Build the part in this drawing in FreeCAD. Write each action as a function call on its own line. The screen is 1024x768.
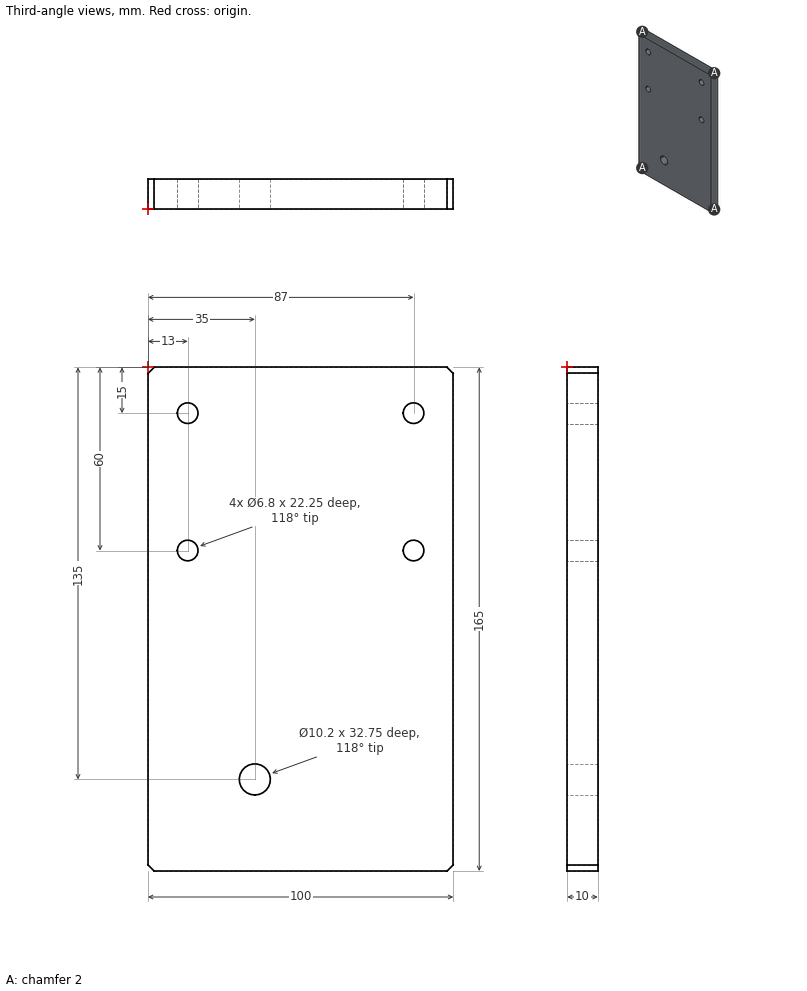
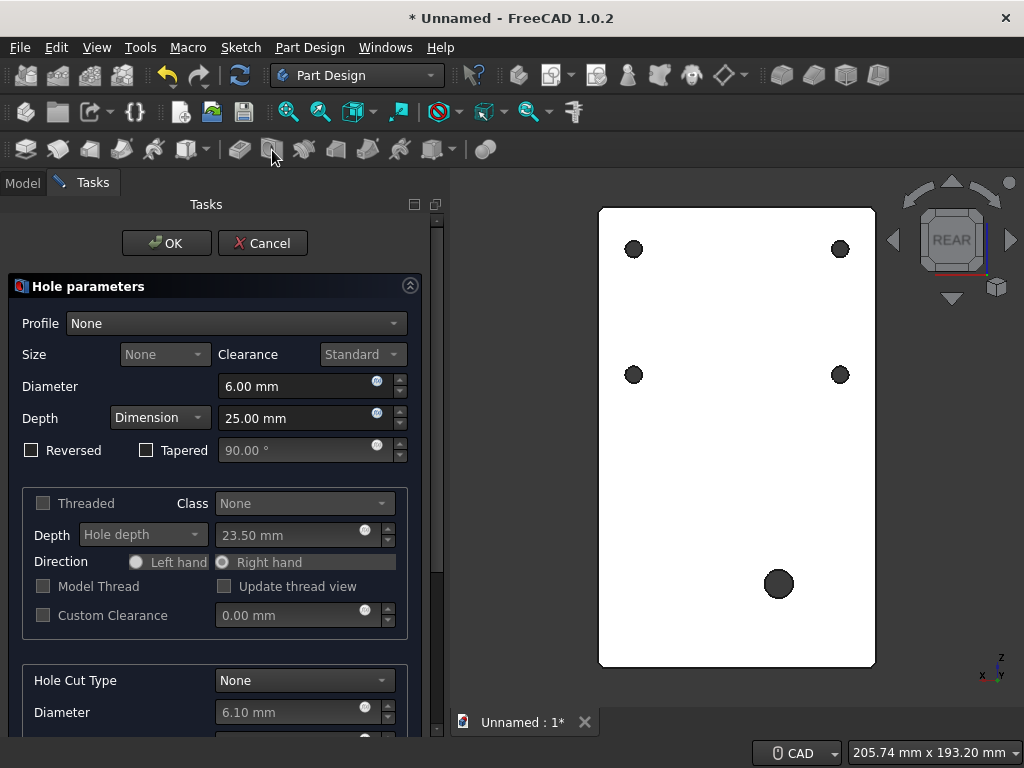
triple_click(305, 386)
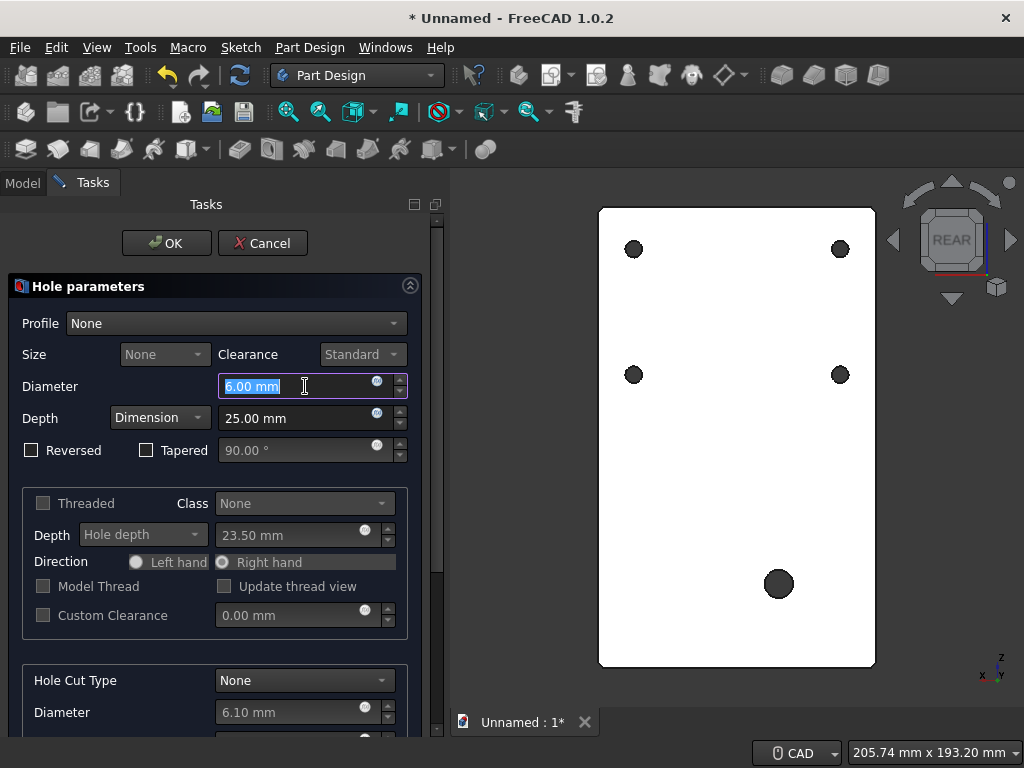
text(6.8)
key(Tab)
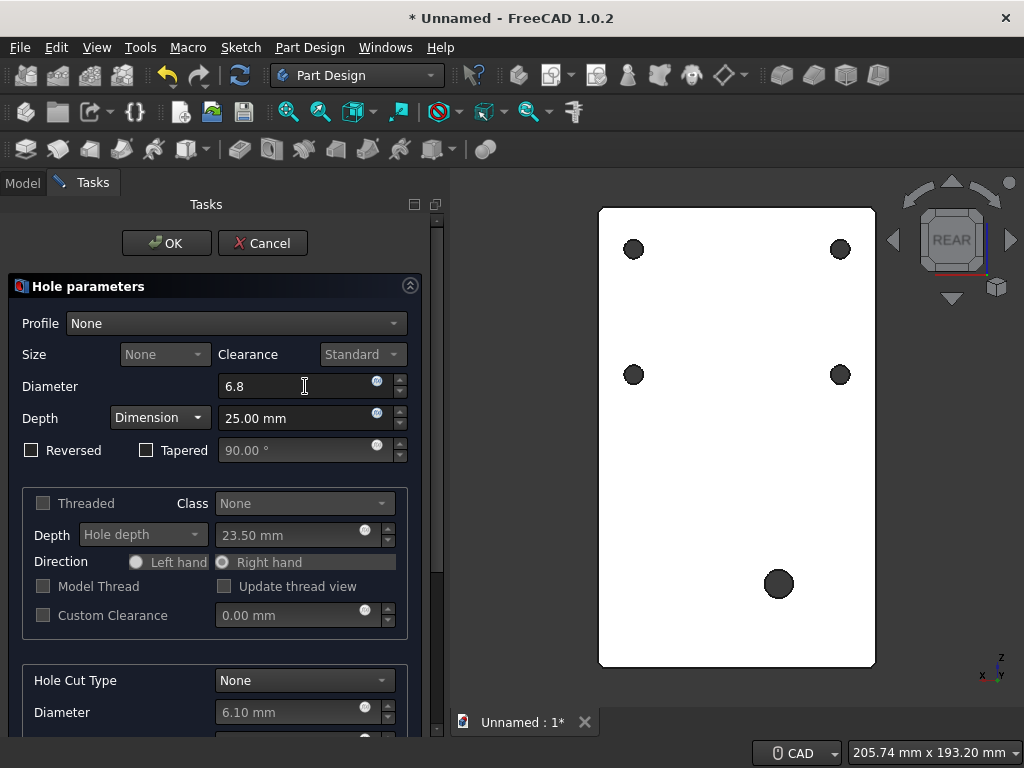
triple_click(305, 418)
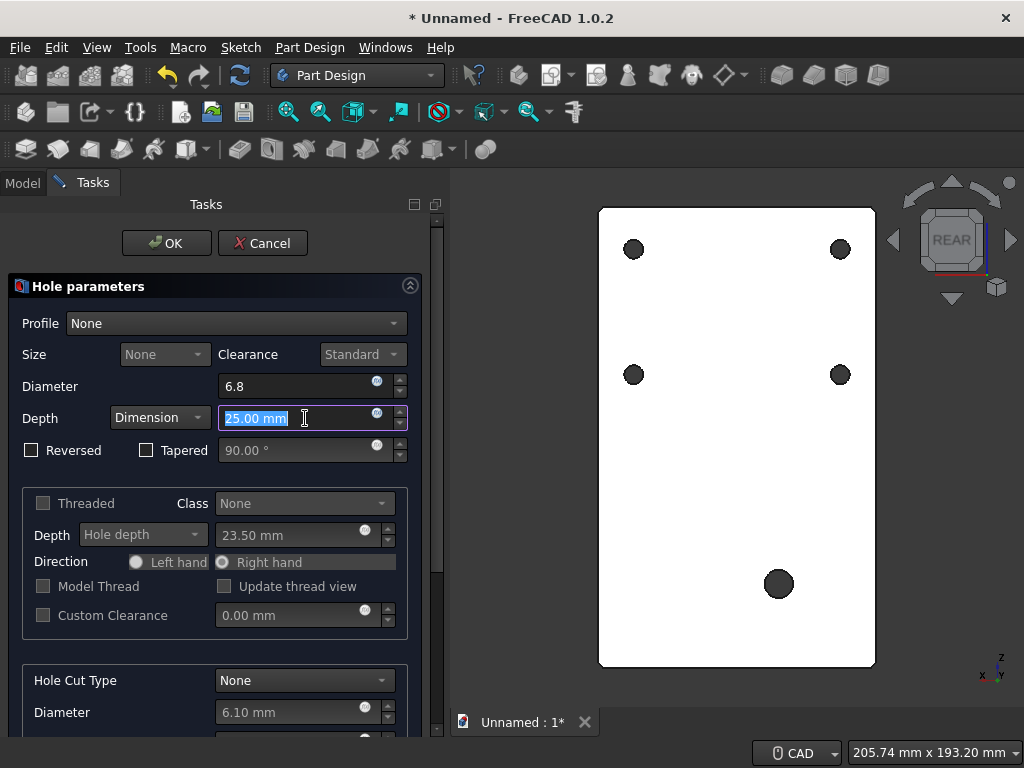
text(22.25)
key(Tab)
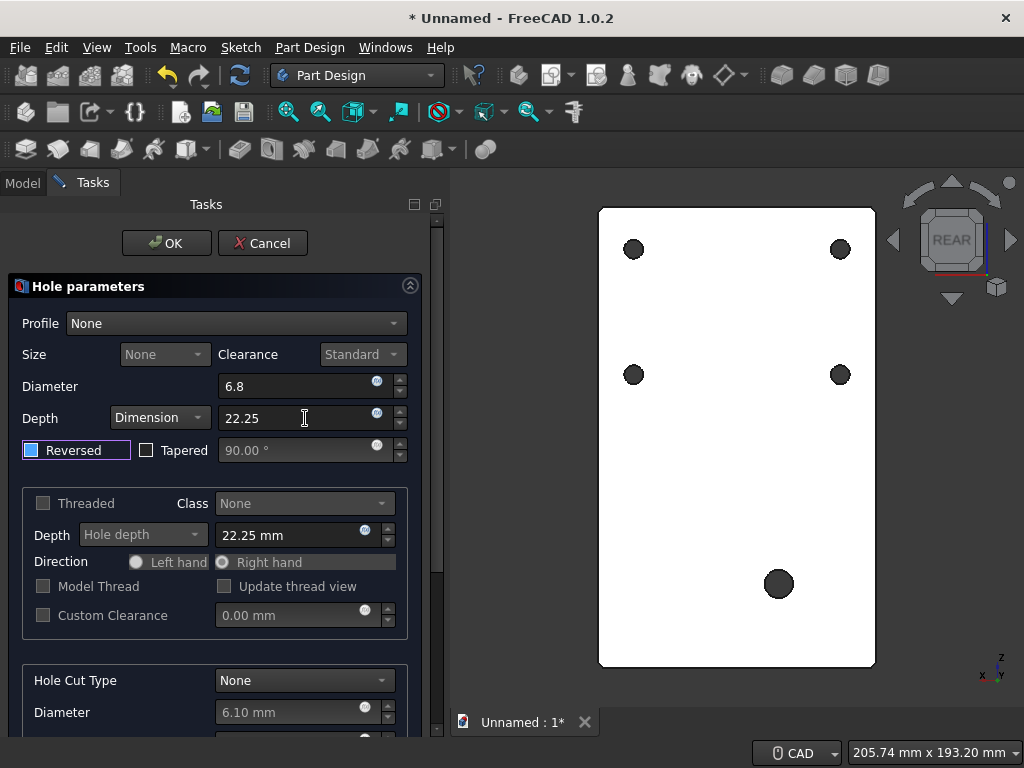
click(167, 243)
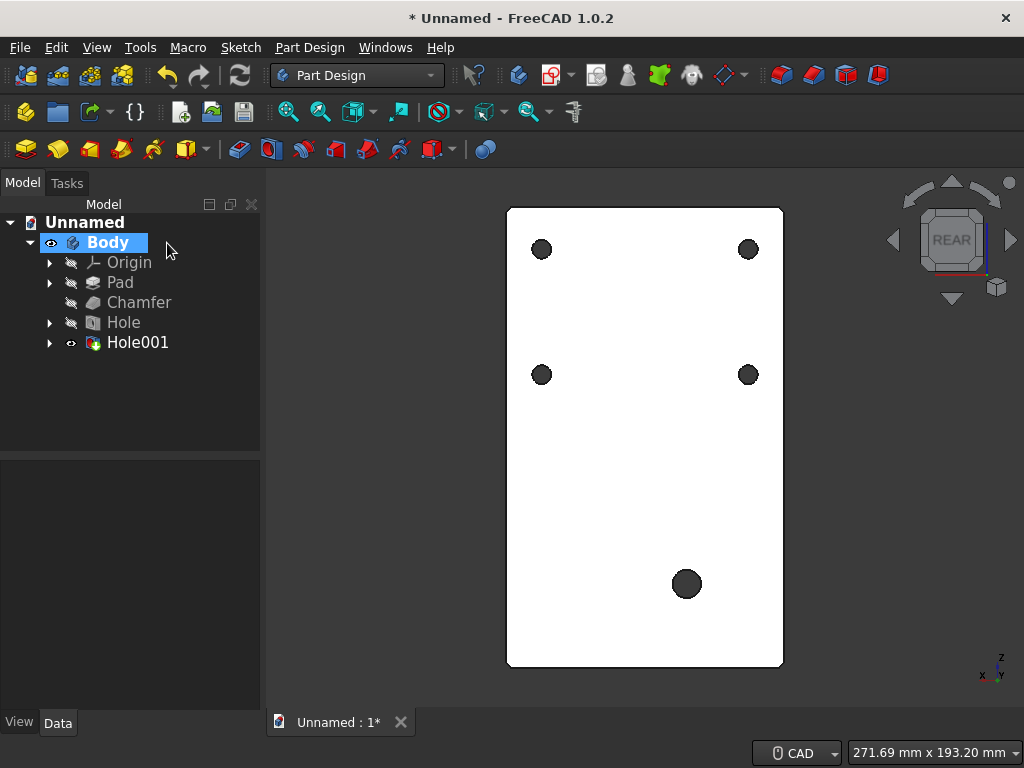
key(0)